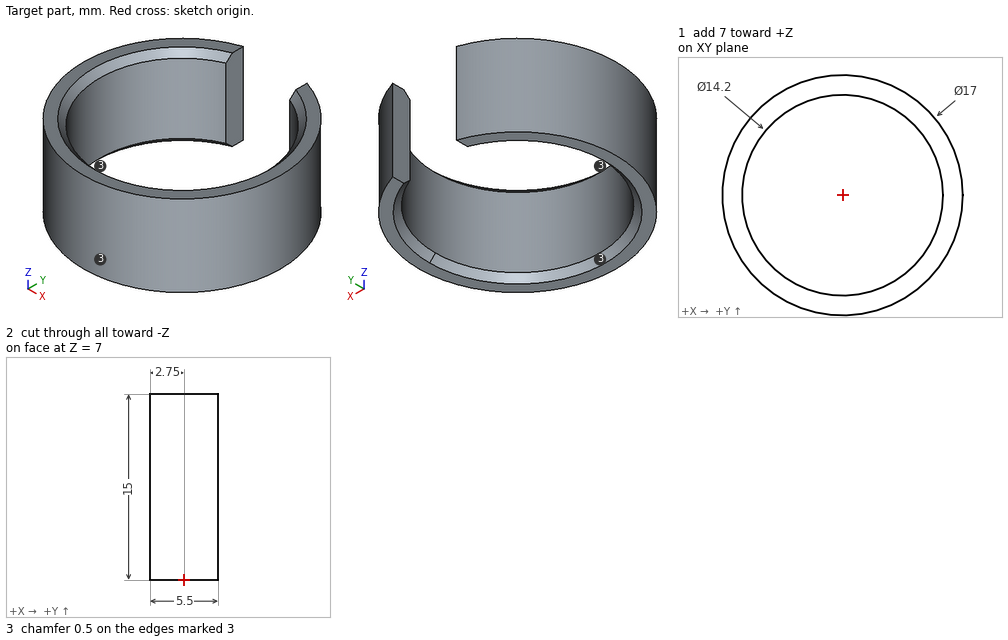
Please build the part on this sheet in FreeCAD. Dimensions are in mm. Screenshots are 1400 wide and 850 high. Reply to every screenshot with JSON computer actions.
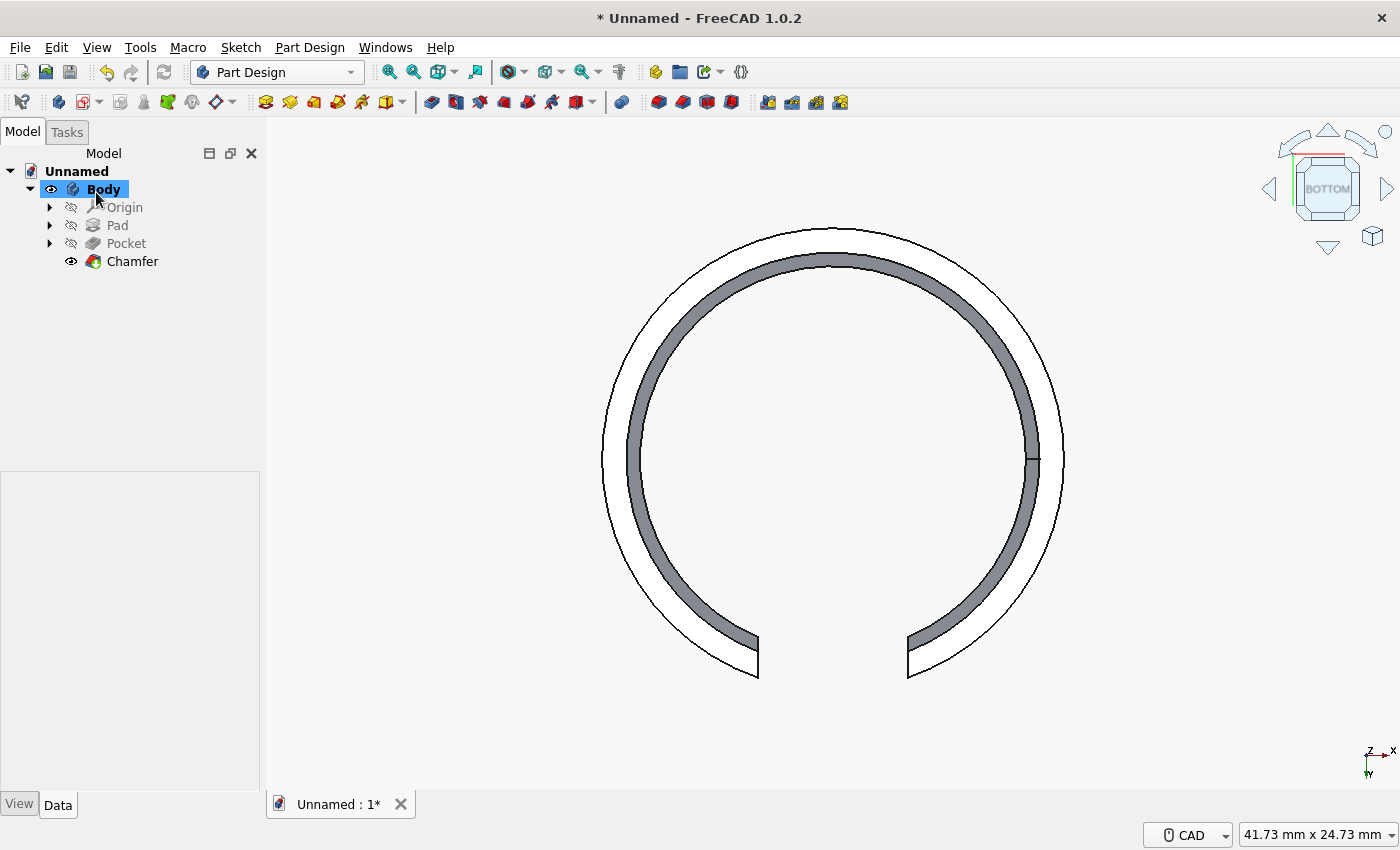
{"action": "key", "text": "0"}